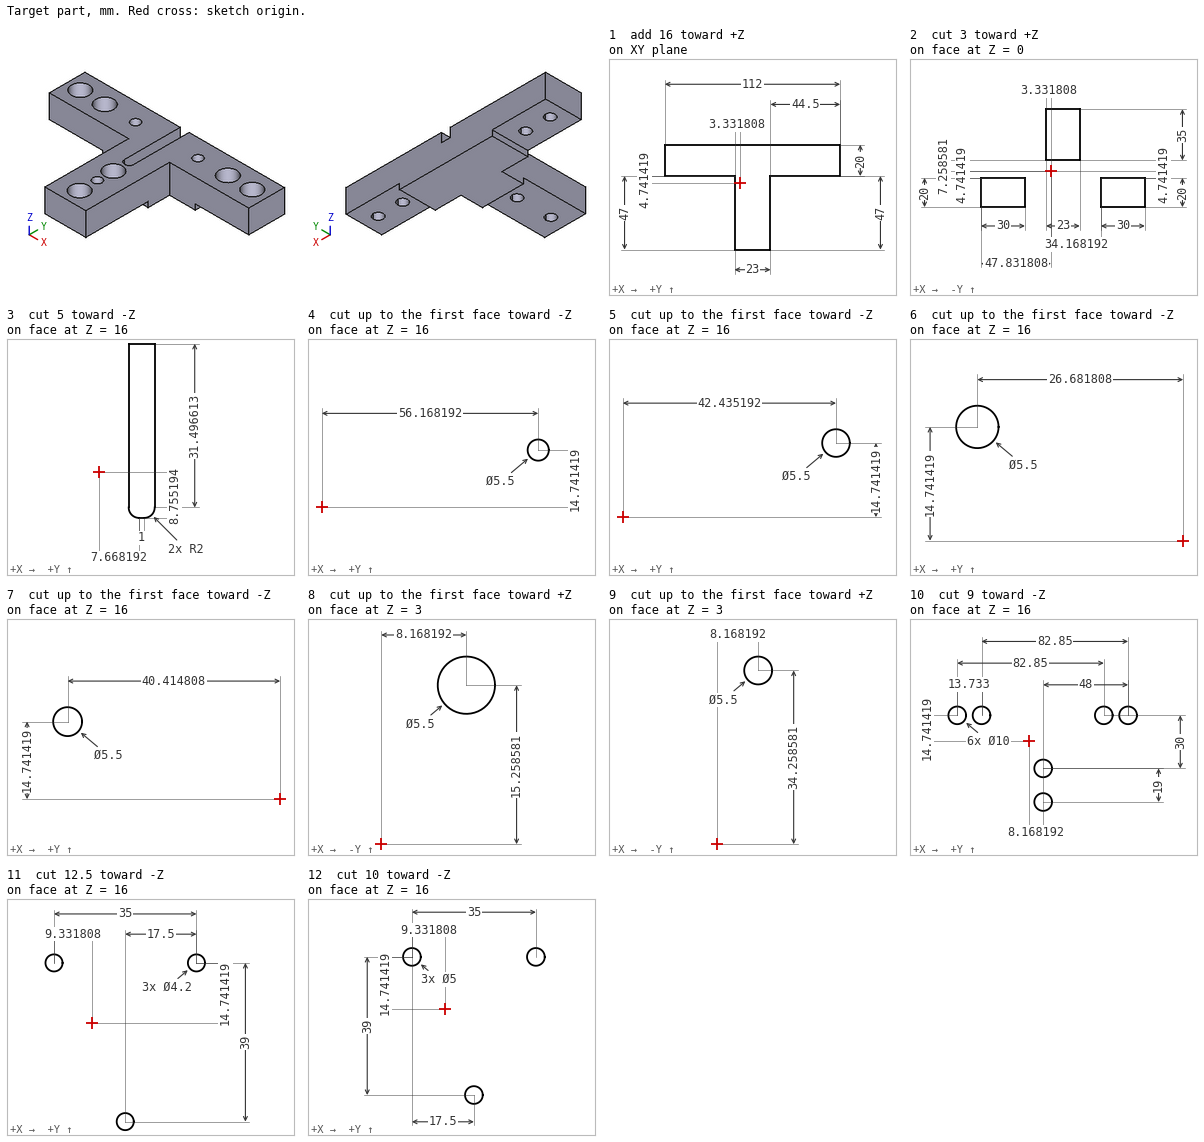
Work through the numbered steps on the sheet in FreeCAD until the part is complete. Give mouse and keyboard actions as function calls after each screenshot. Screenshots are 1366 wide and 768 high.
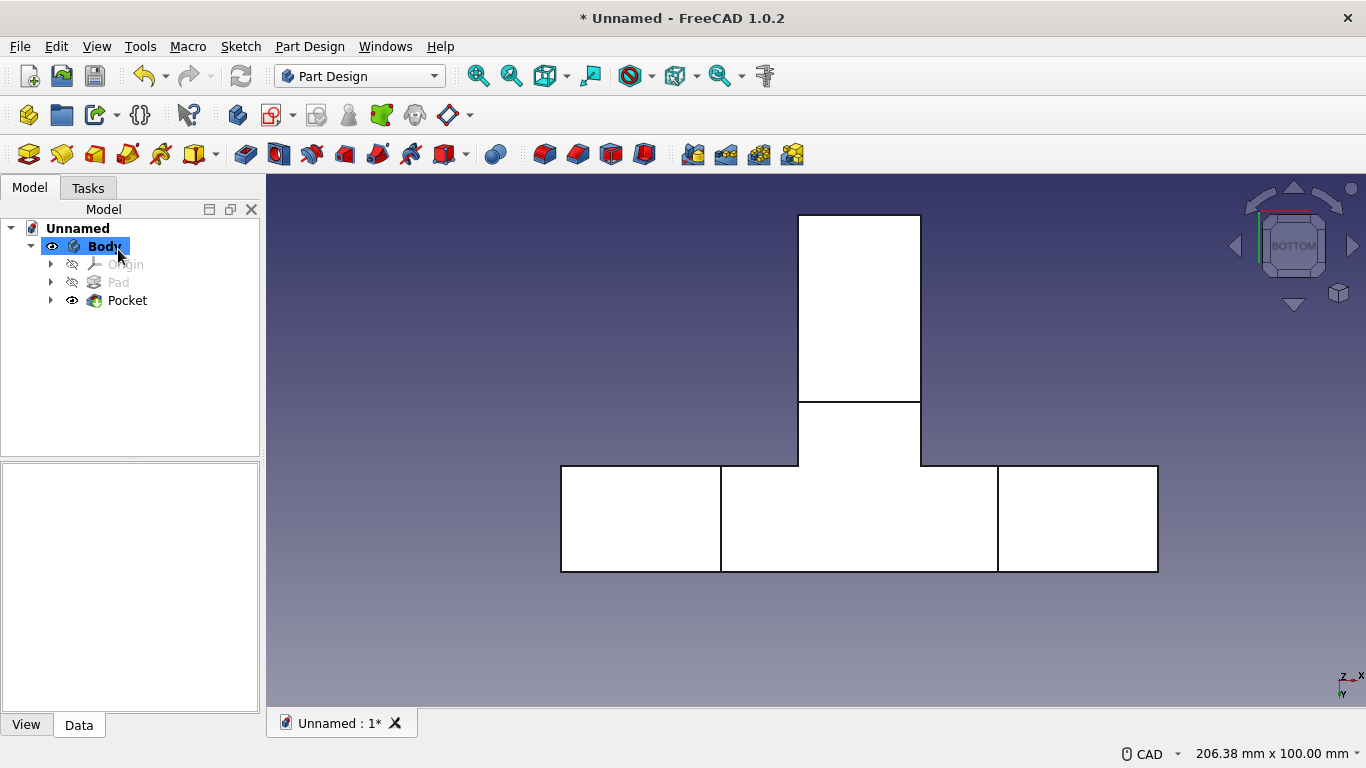
key(0)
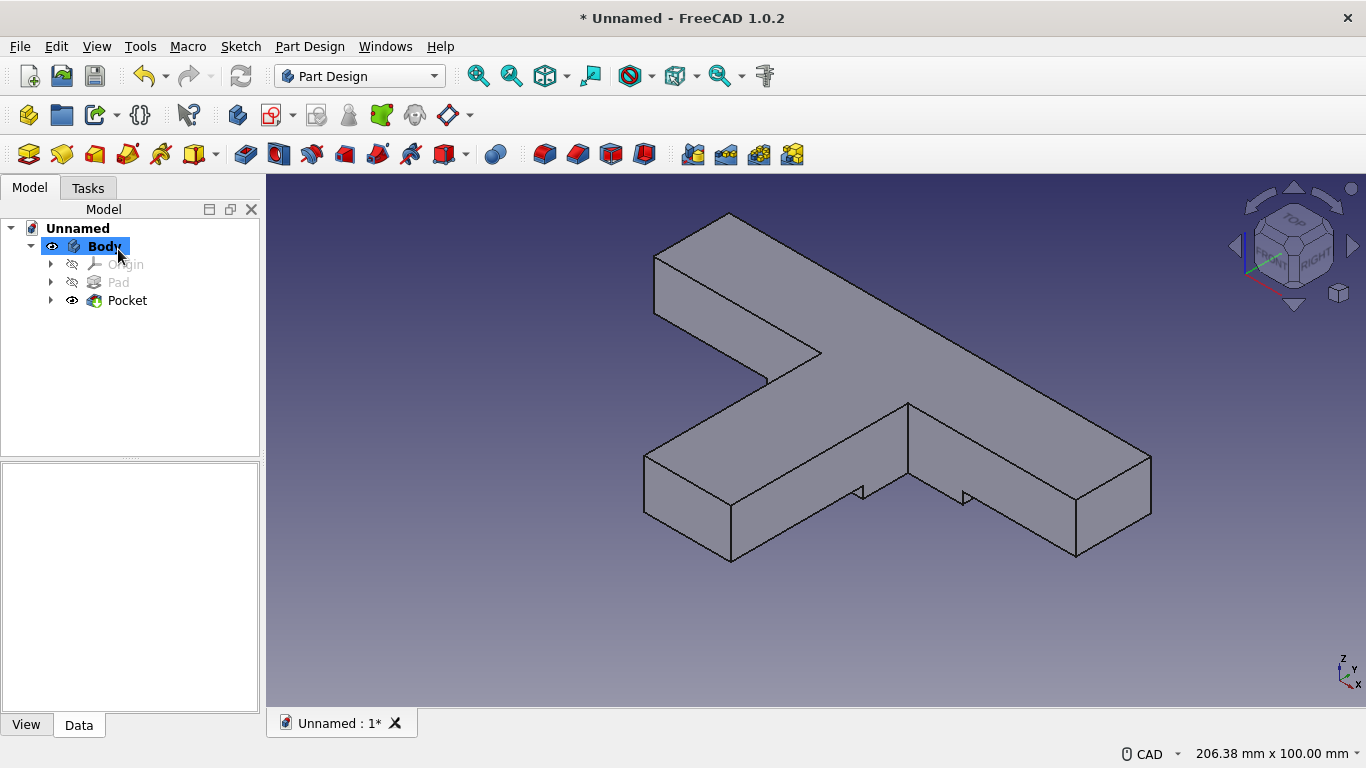
click(886, 365)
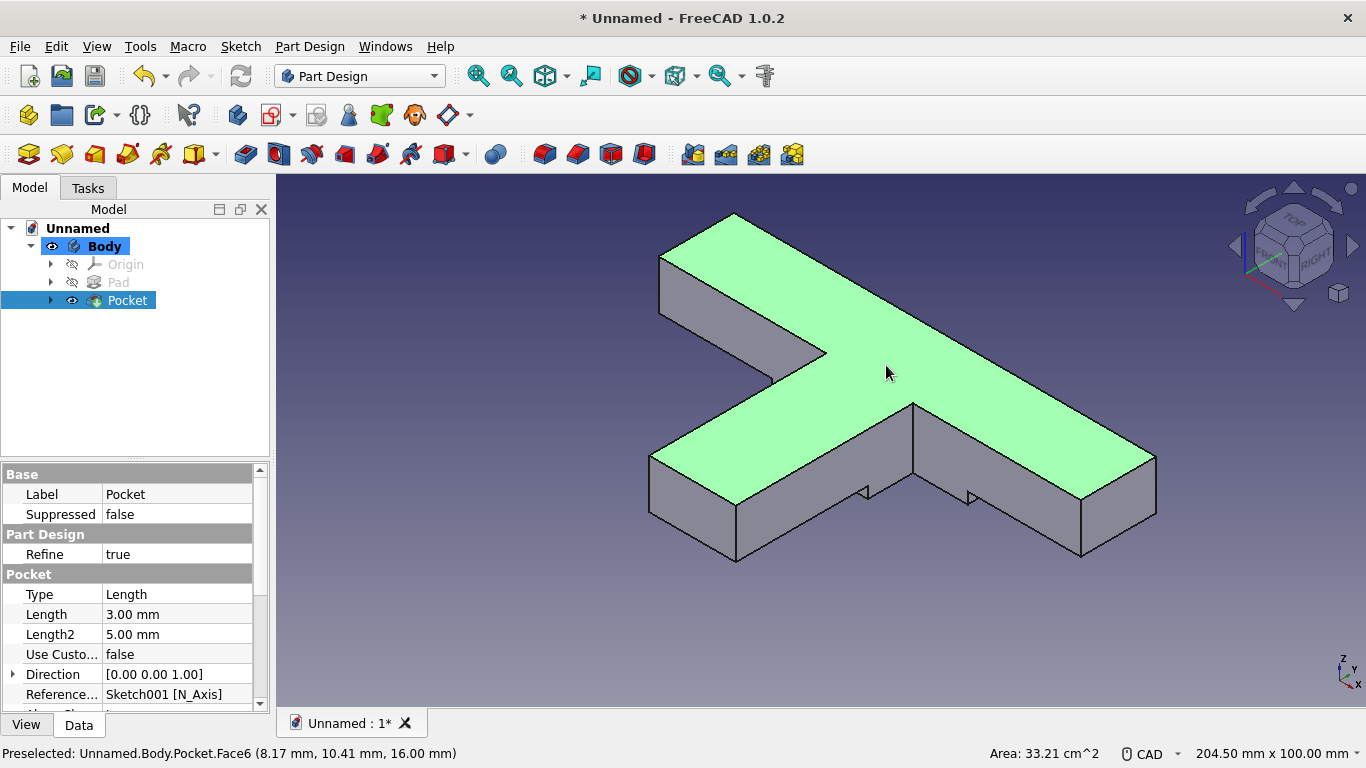
click(270, 116)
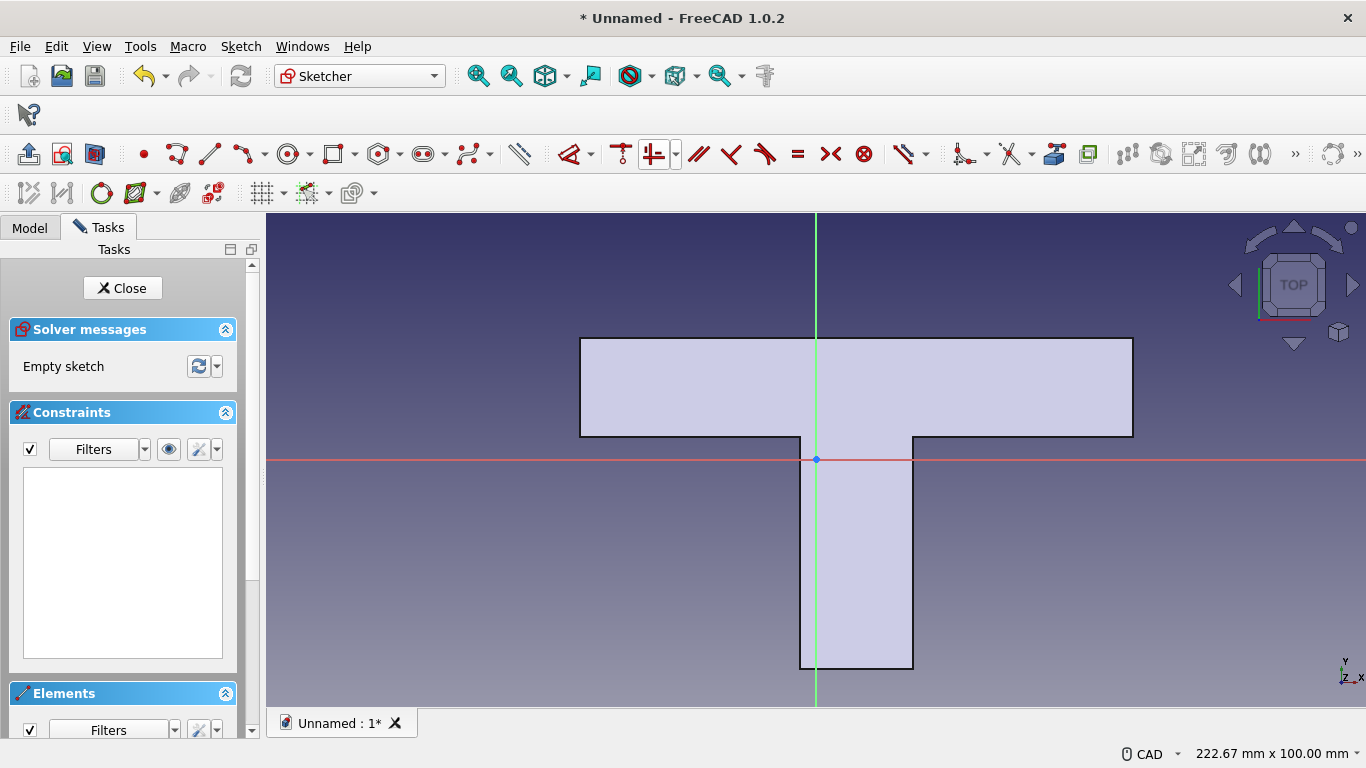
scroll(958, 372, up, 3)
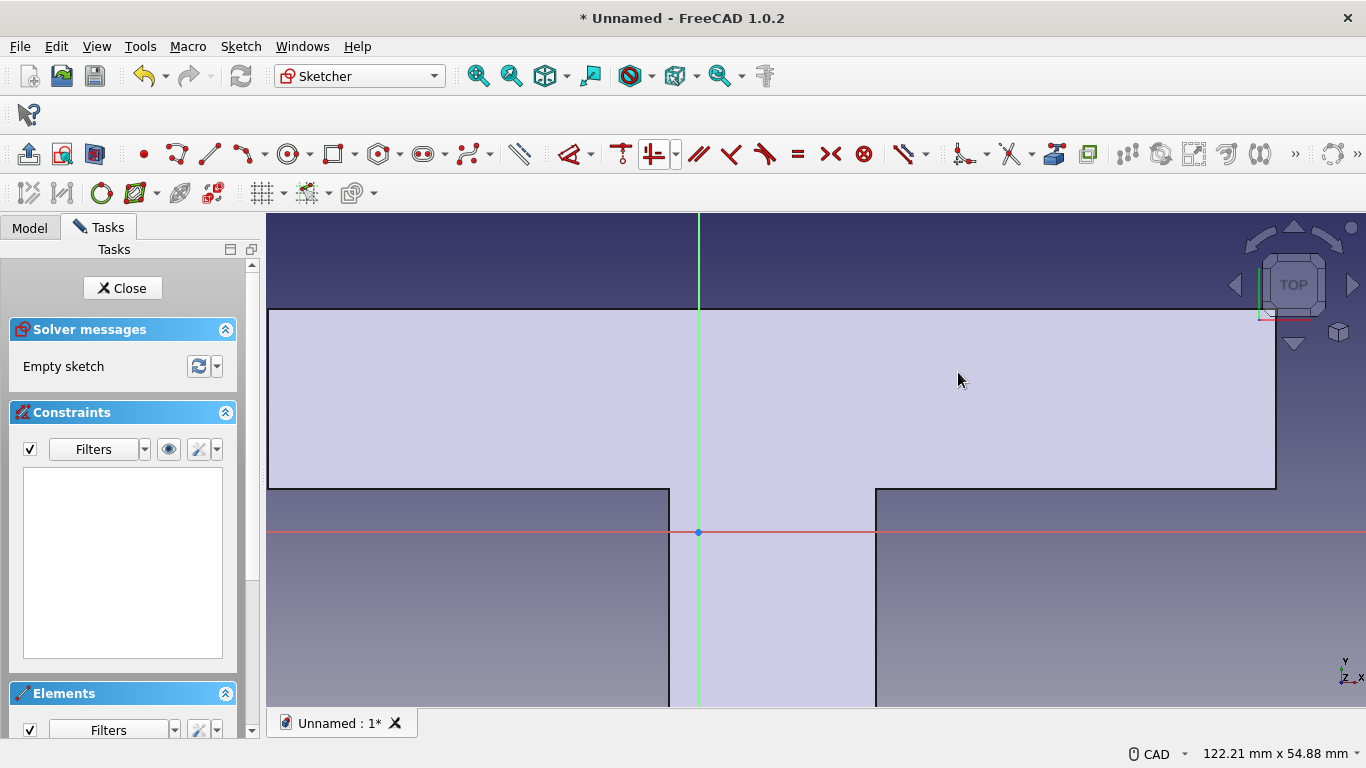
click(210, 154)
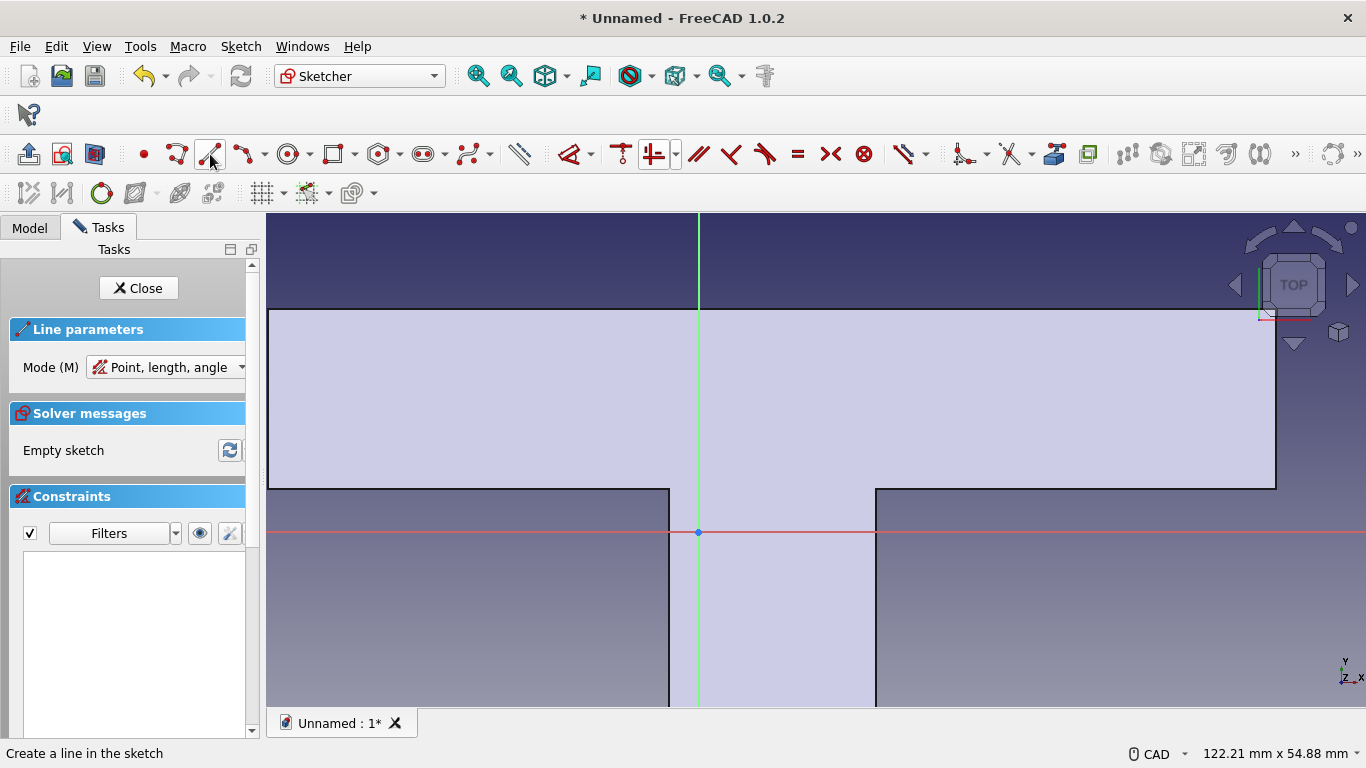
click(768, 611)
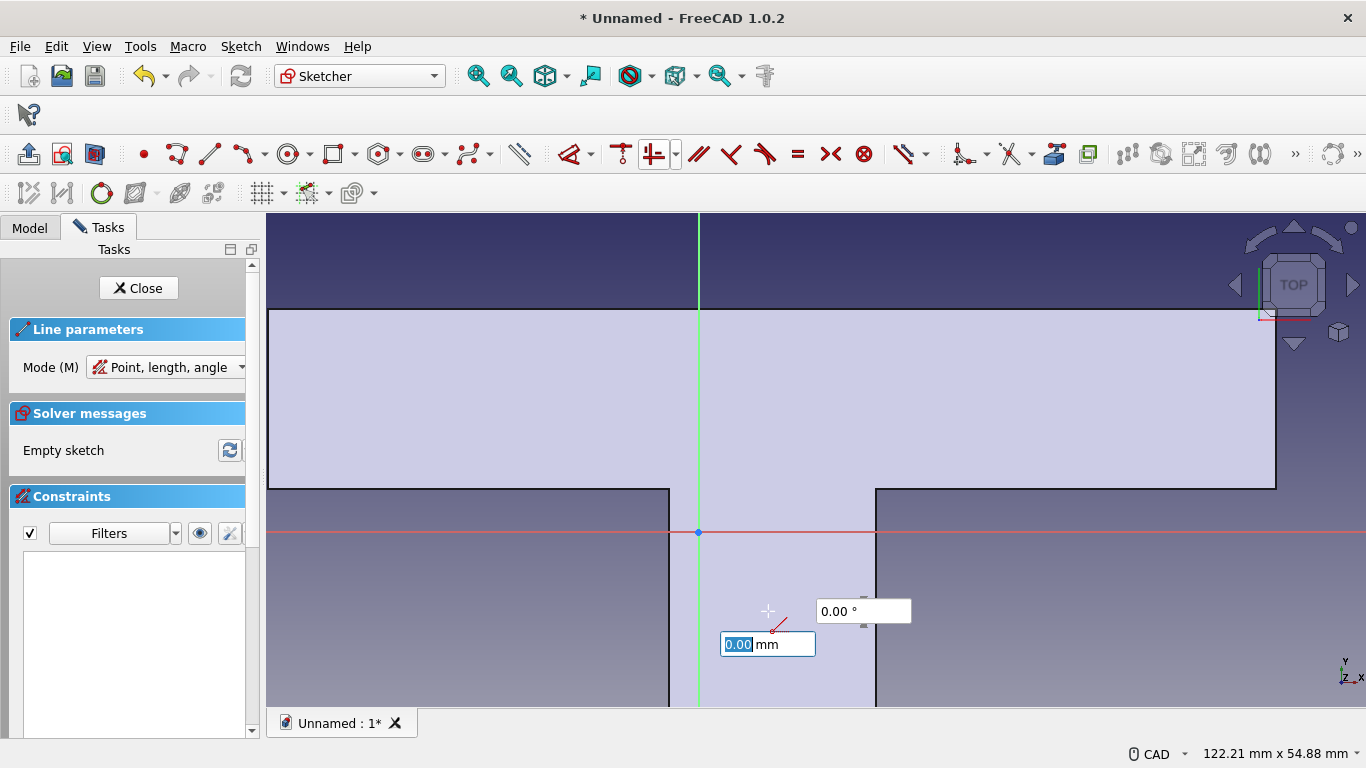
scroll(777, 611, up, 3)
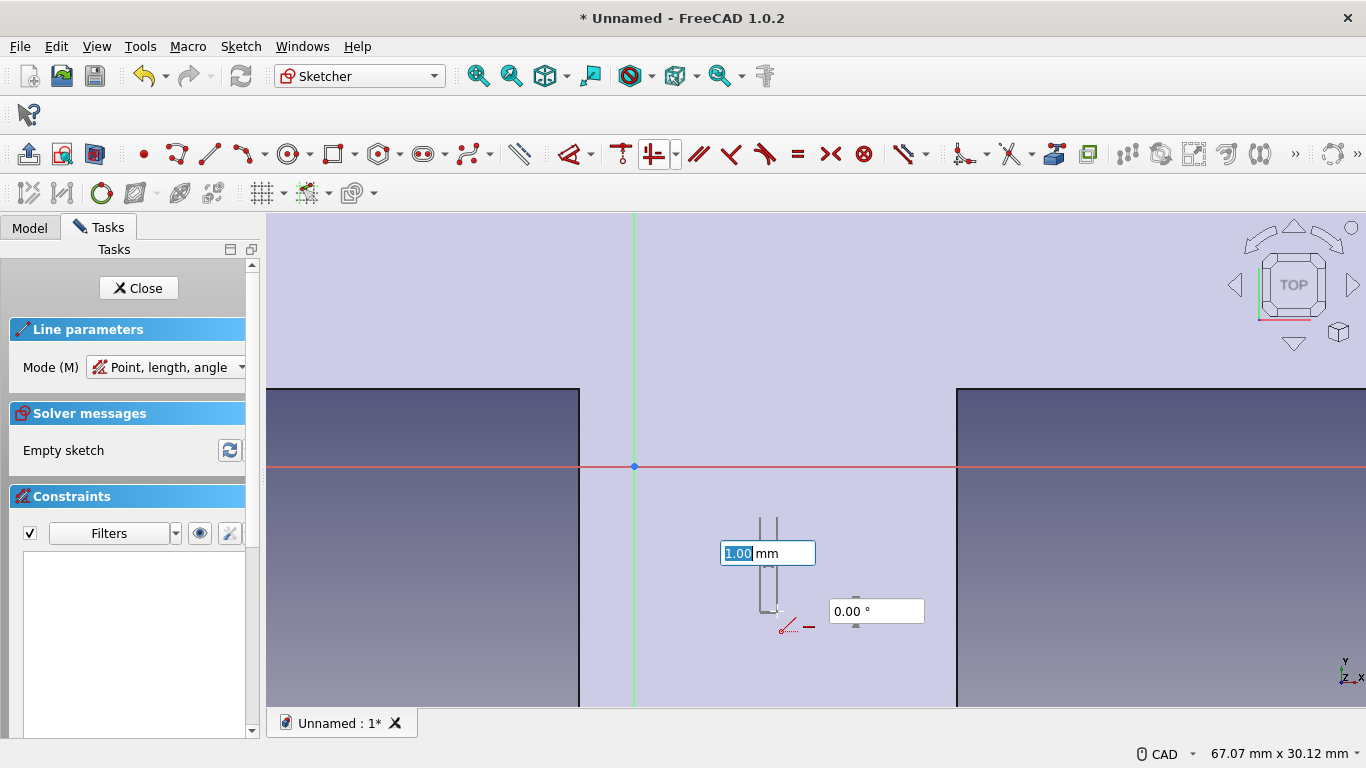
click(776, 610)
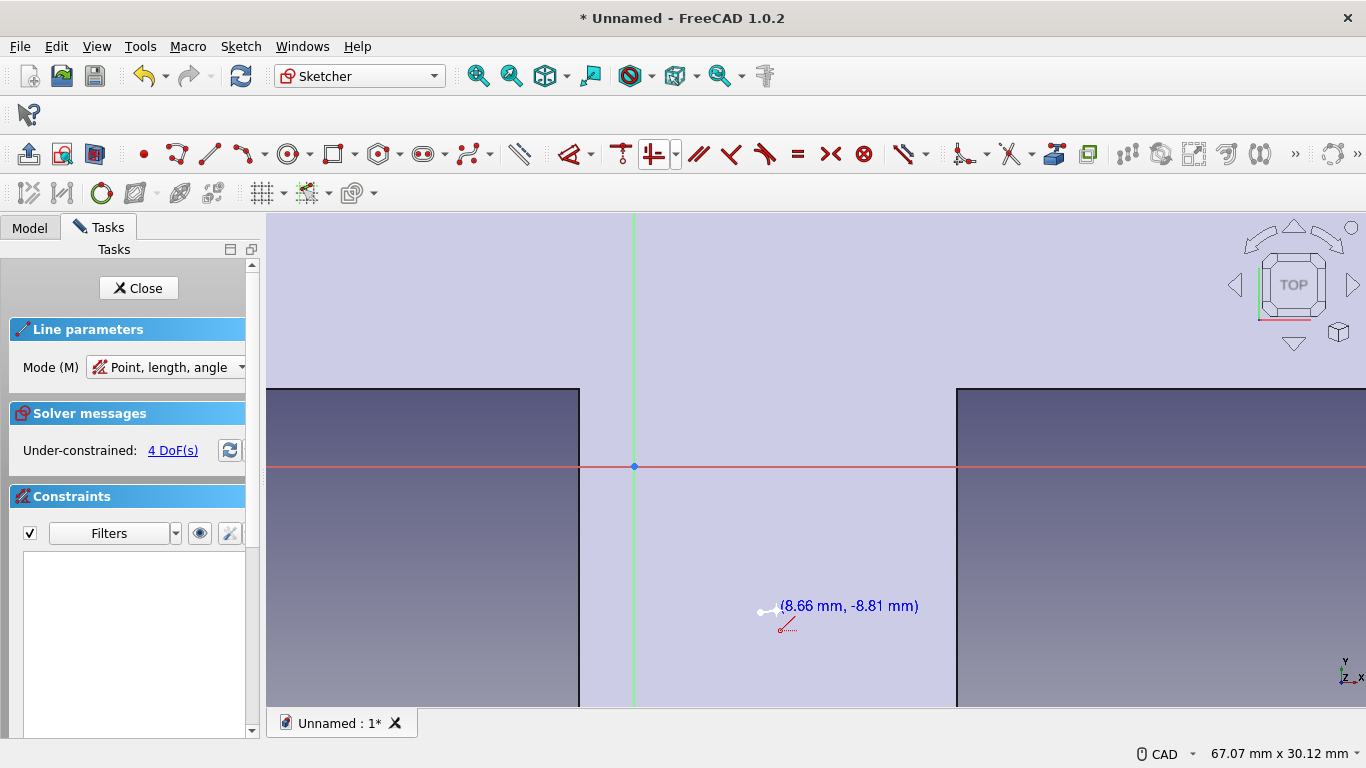
key(g)
key(m)